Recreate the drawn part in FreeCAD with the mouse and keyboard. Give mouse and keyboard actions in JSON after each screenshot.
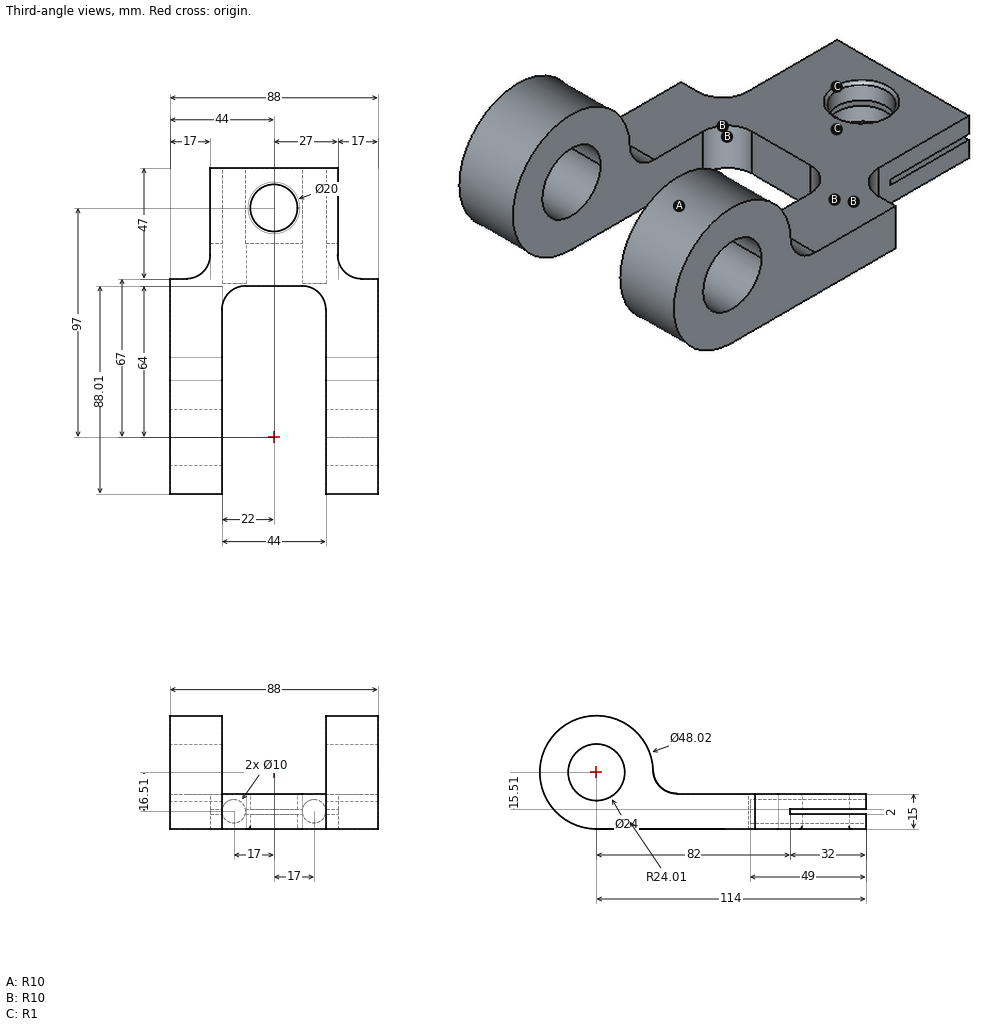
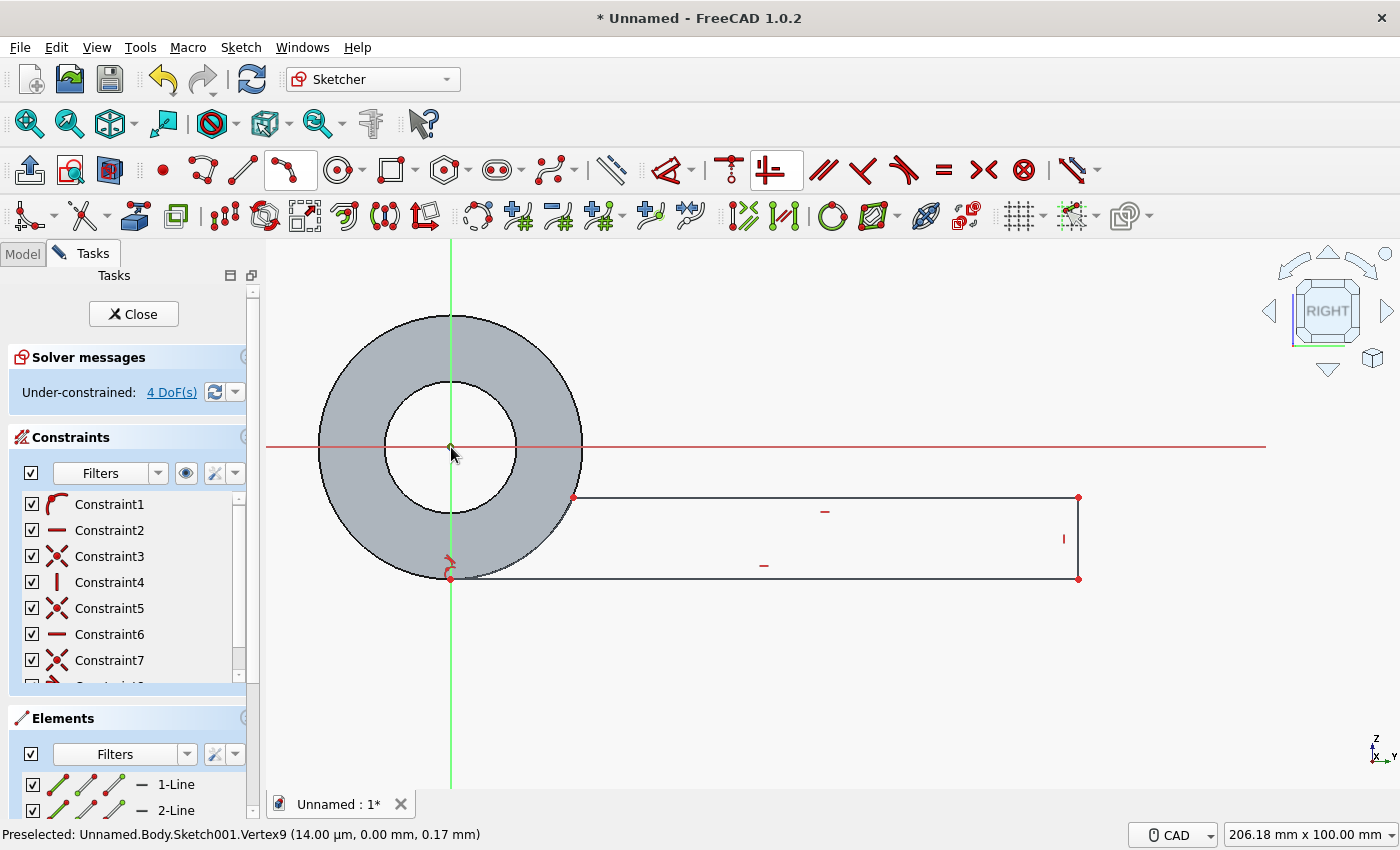
{"action": "left_click", "coordinate": [361, 447]}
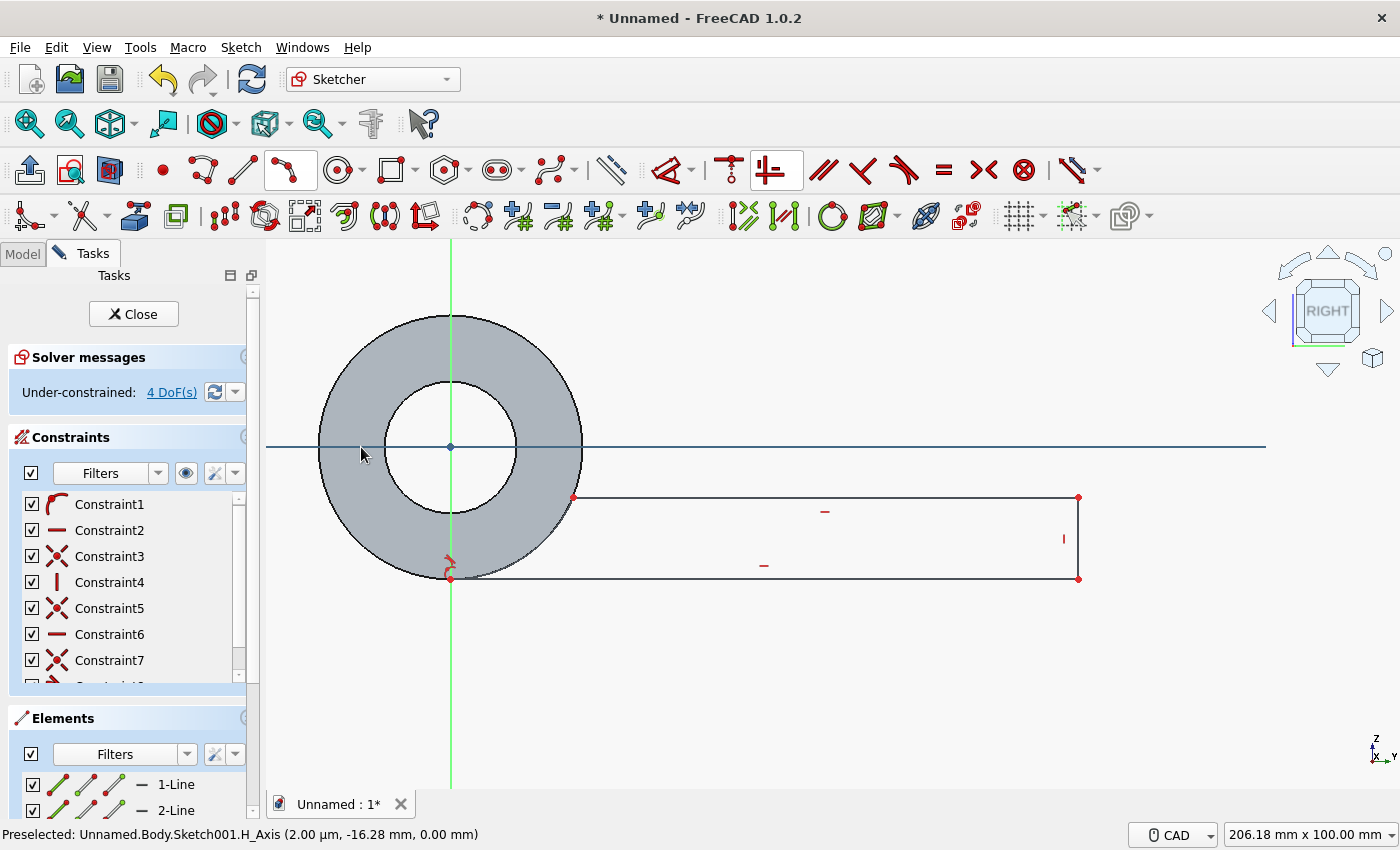
{"action": "left_click", "coordinate": [730, 170]}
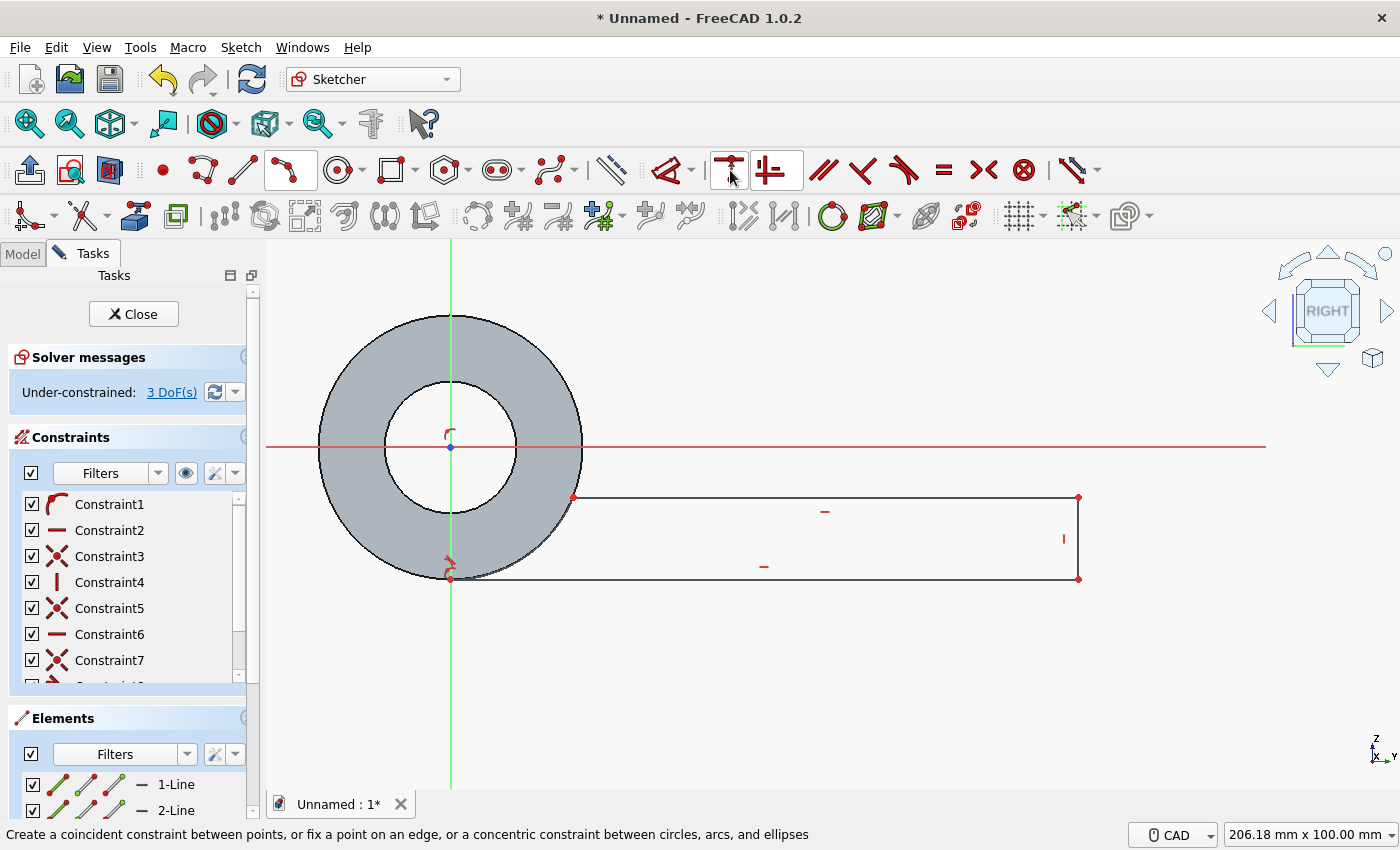
{"action": "left_click", "coordinate": [666, 170]}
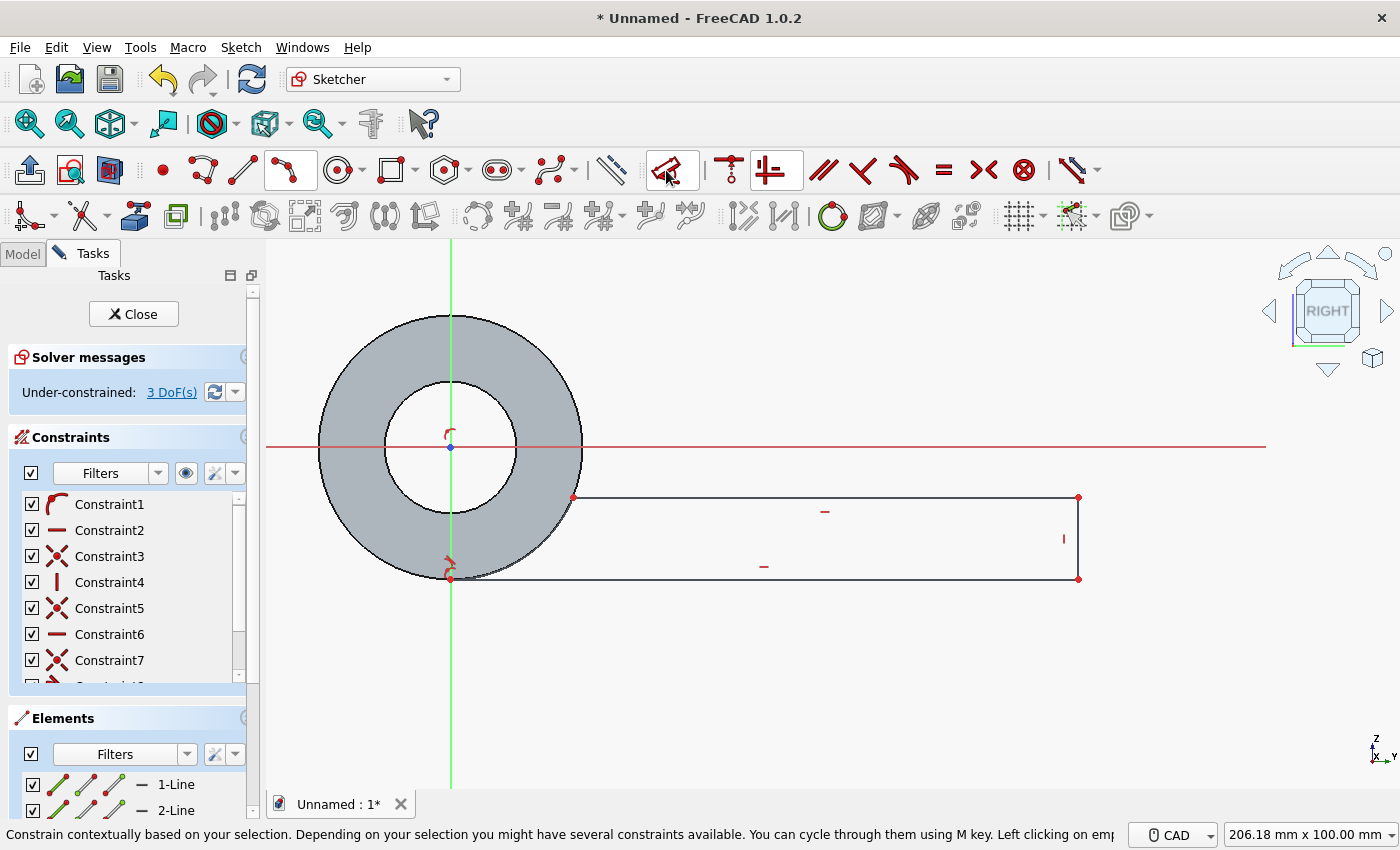
{"action": "left_click", "coordinate": [548, 537]}
{"action": "left_click", "coordinate": [572, 559]}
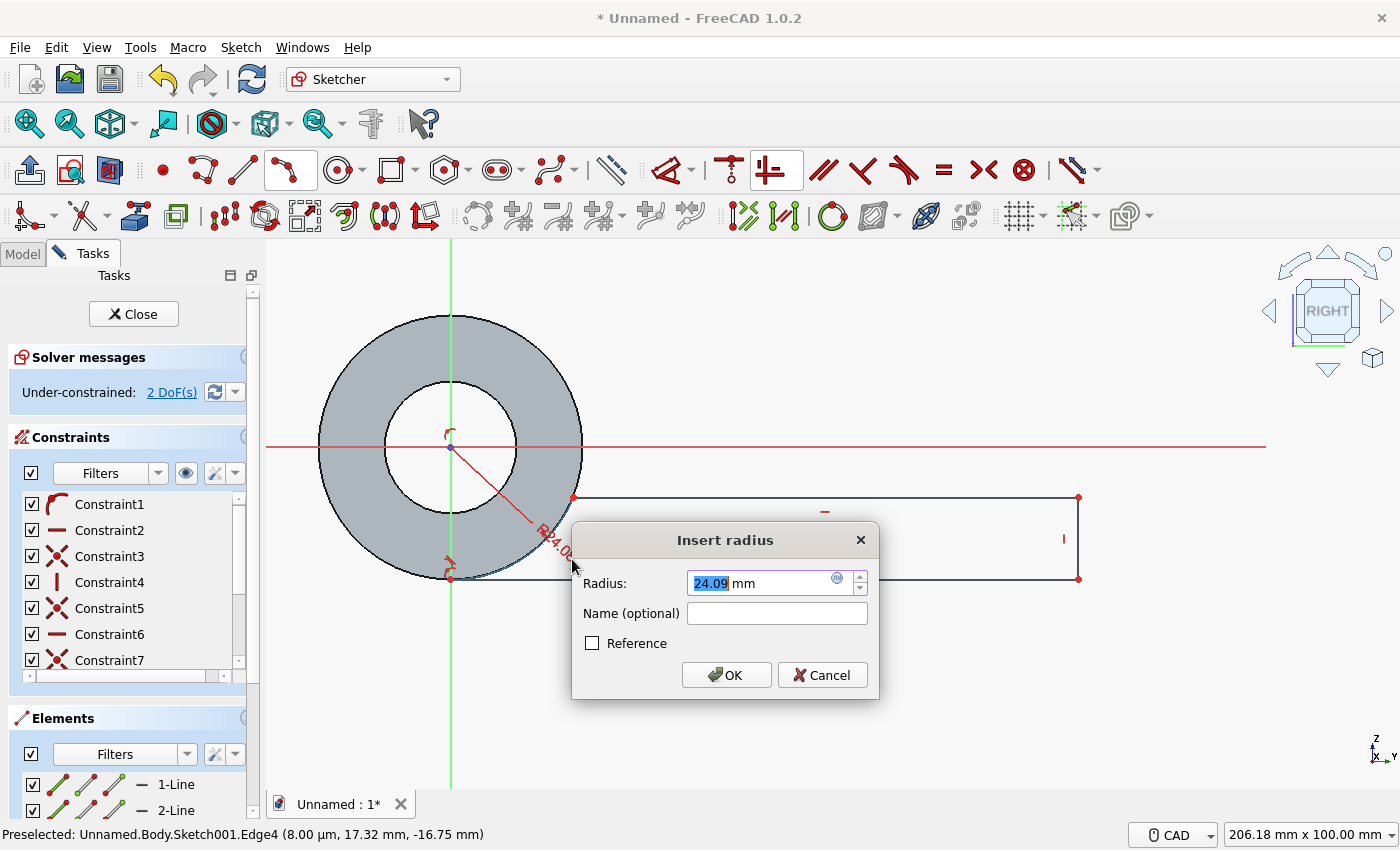
{"action": "type", "text": "24.01"}
{"action": "key", "text": "Return"}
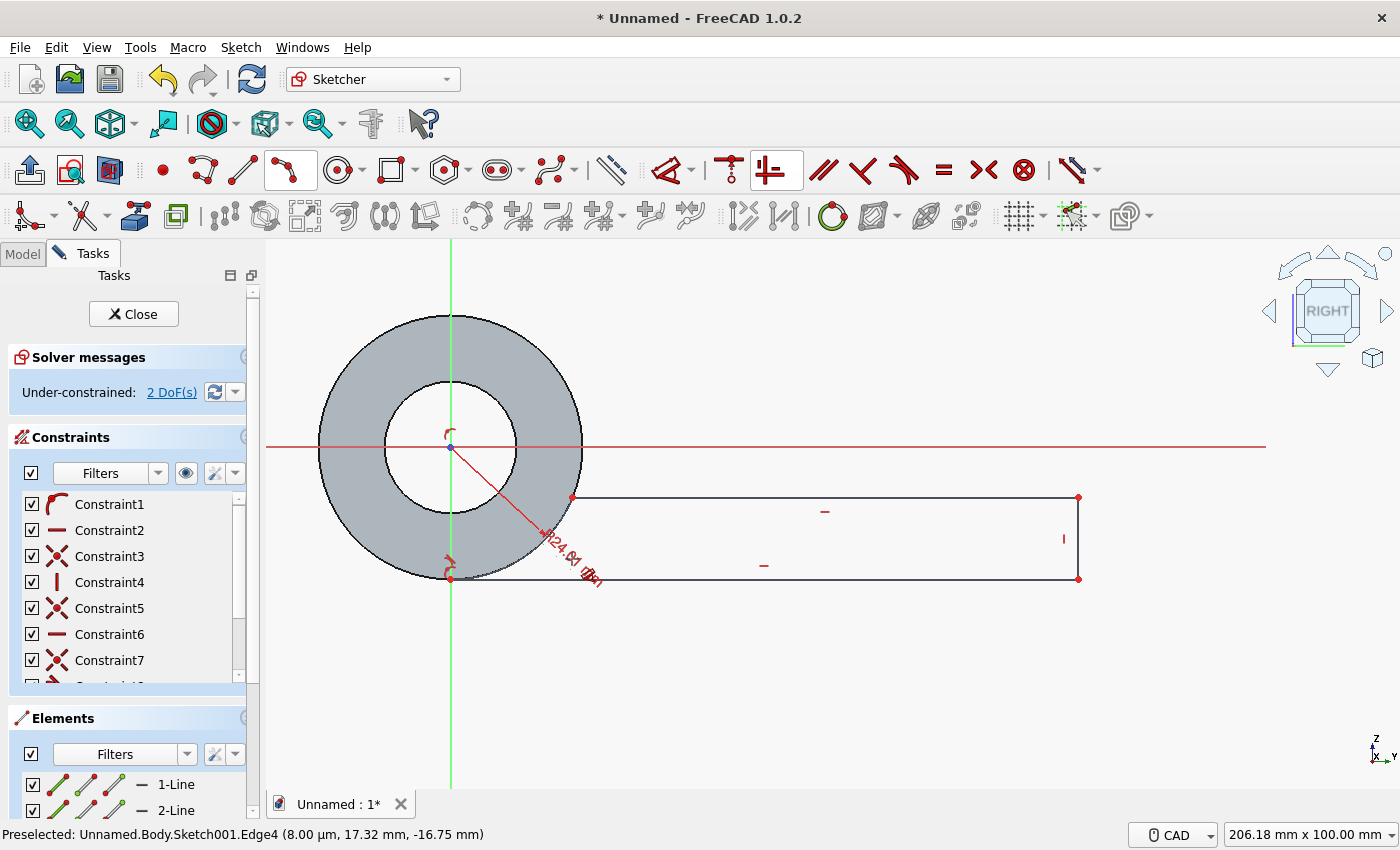
{"action": "left_click", "coordinate": [1078, 555]}
{"action": "left_click", "coordinate": [1112, 539]}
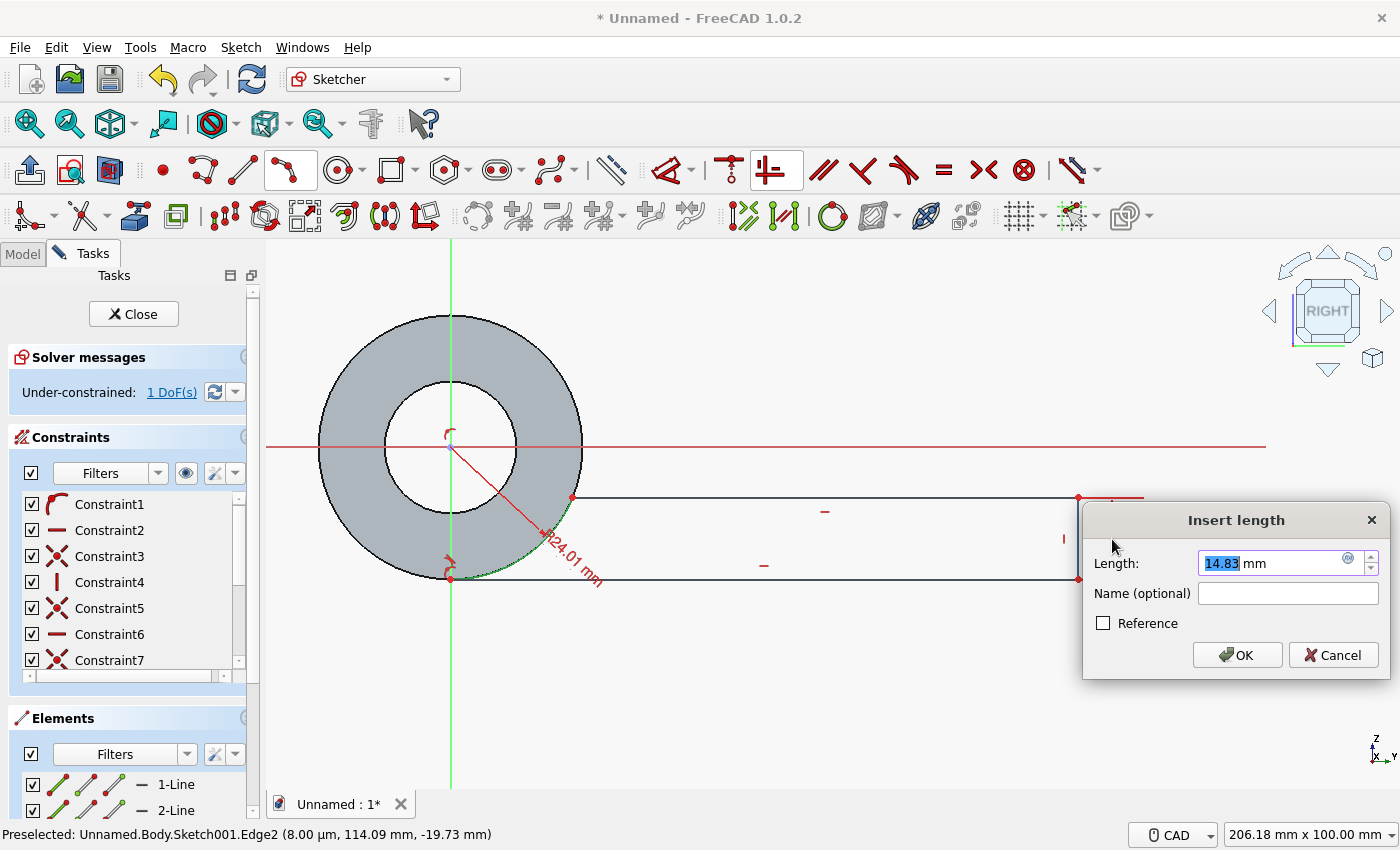
{"action": "type", "text": "15"}
{"action": "key", "text": "Return"}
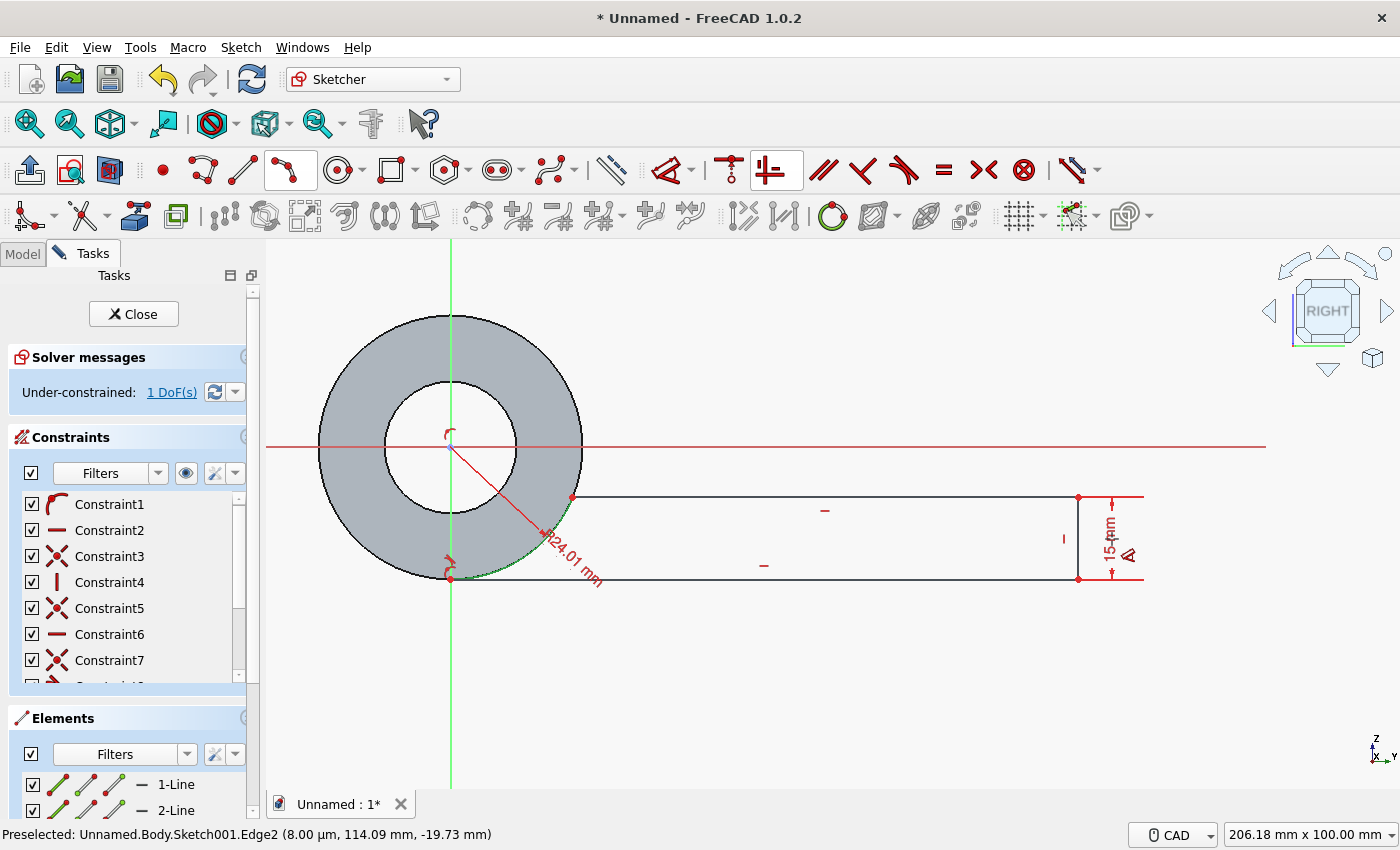
{"action": "left_click", "coordinate": [639, 580]}
{"action": "left_click", "coordinate": [764, 614]}